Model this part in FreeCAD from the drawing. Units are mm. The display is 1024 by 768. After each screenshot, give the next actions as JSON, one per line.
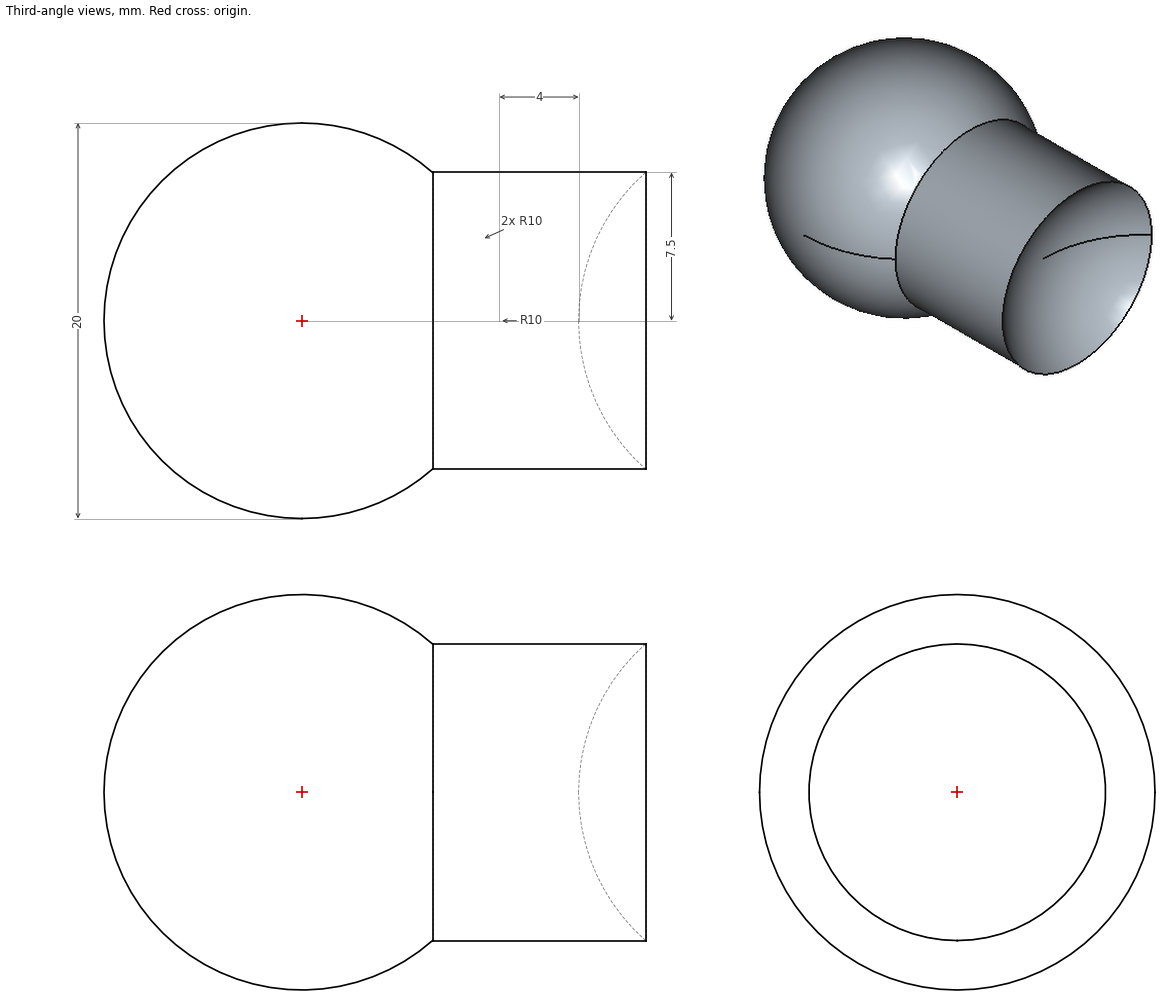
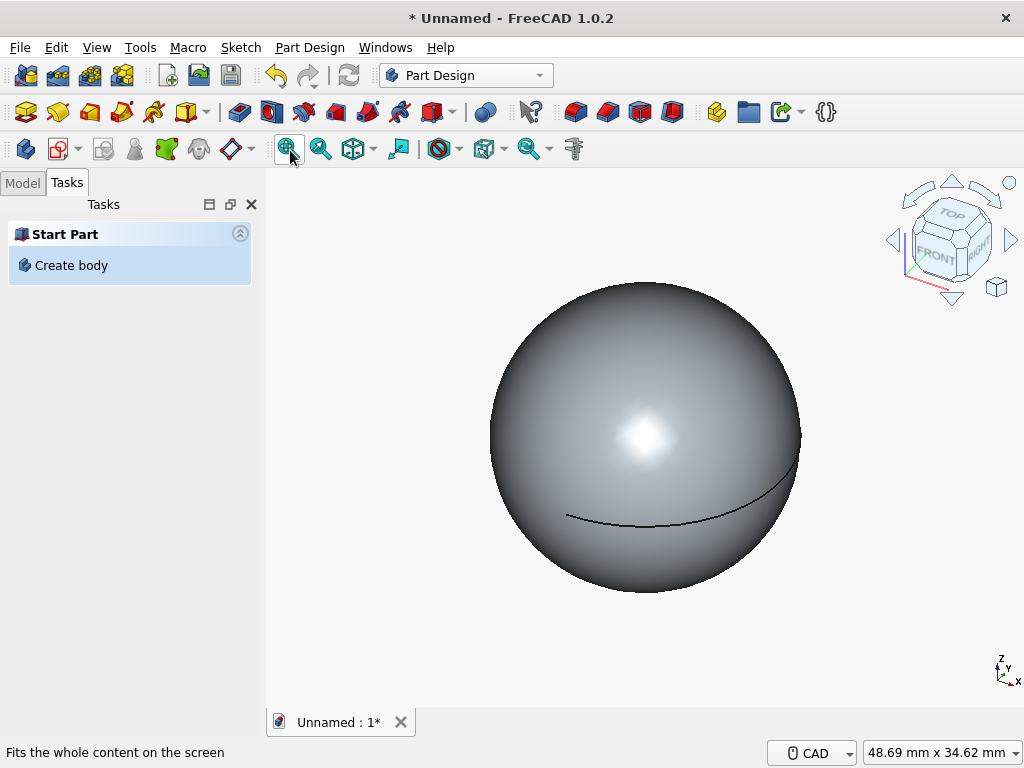
{"action": "left_click", "coordinate": [58, 150]}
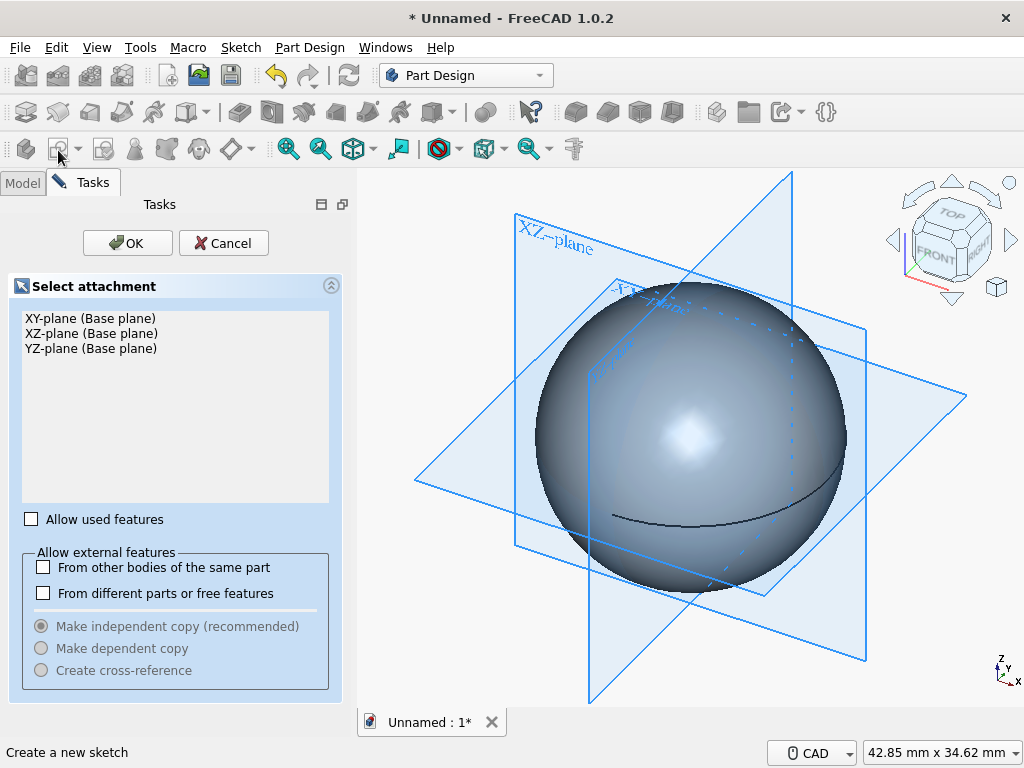
{"action": "left_click", "coordinate": [82, 318]}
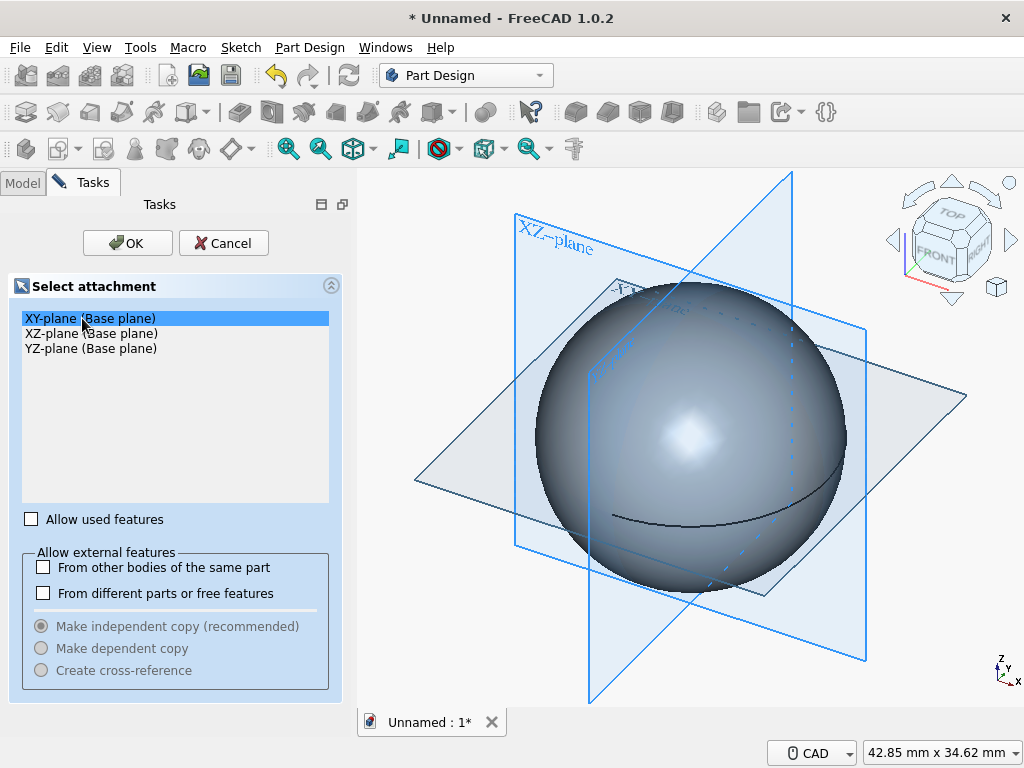
{"action": "left_click", "coordinate": [128, 243]}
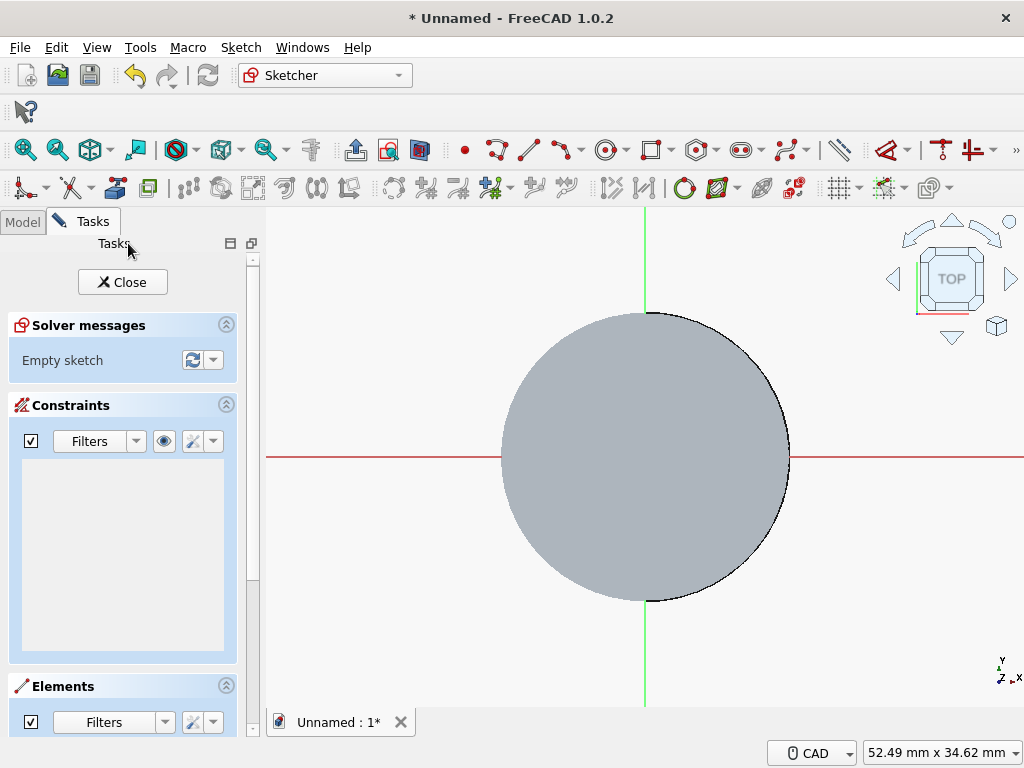
{"action": "key", "text": "q s"}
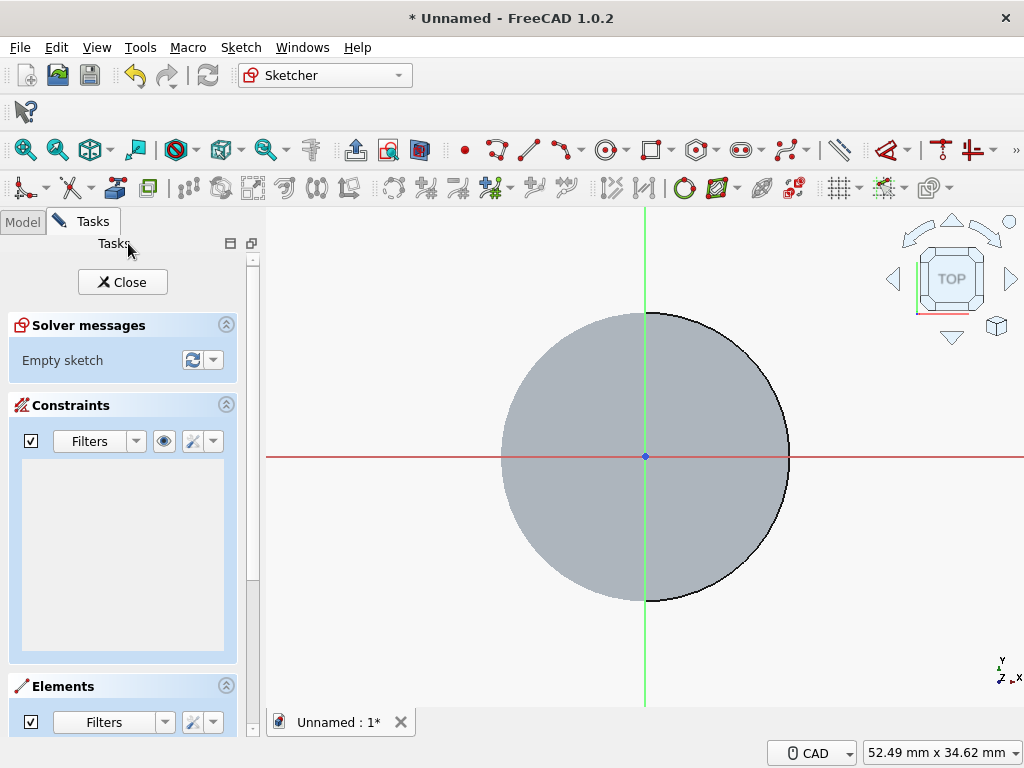
{"action": "scroll", "coordinate": [294, 679], "scroll_direction": "down", "scroll_amount": 1}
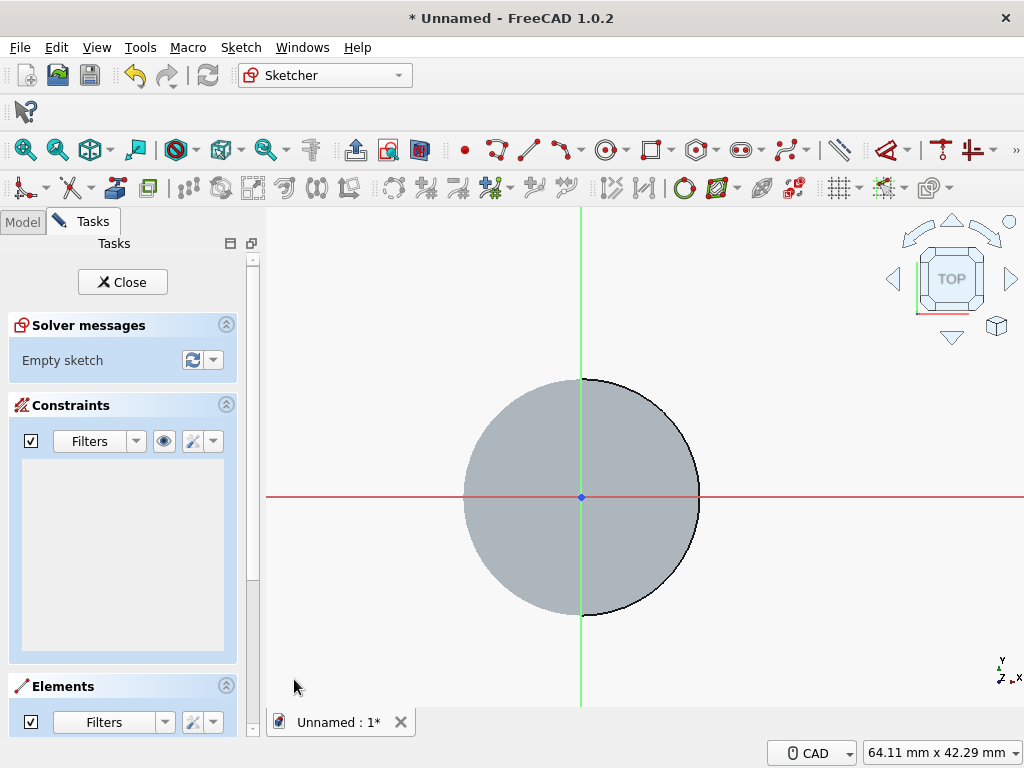
{"action": "scroll", "coordinate": [815, 448], "scroll_direction": "up", "scroll_amount": 3}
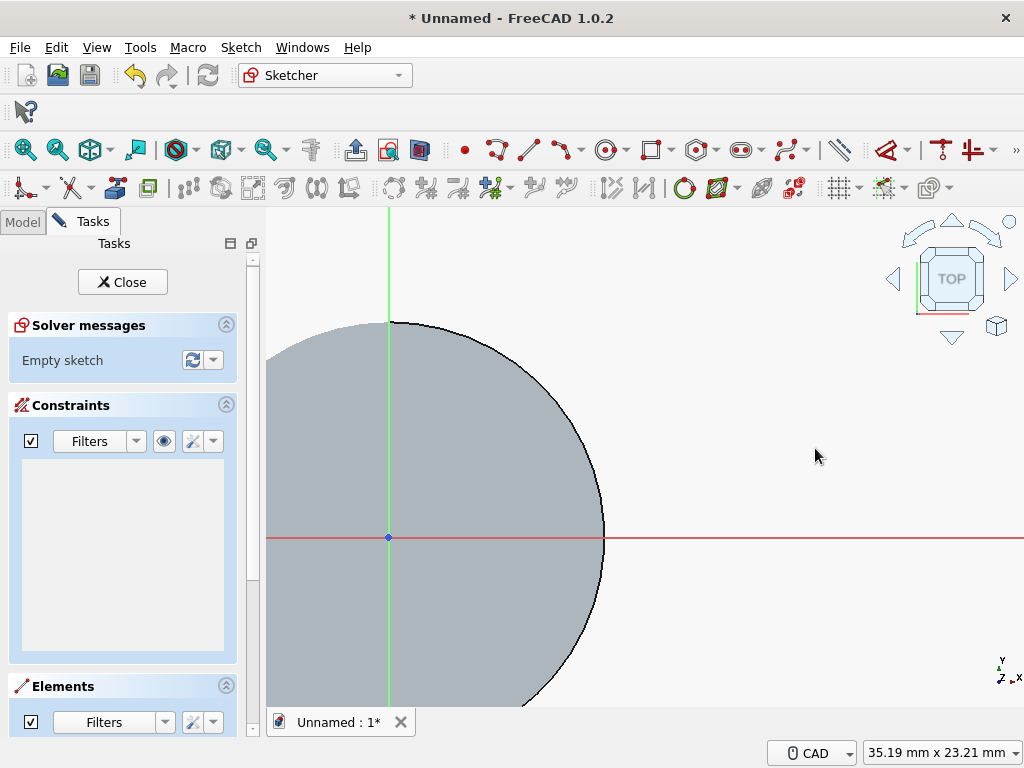
{"action": "key", "text": "g l"}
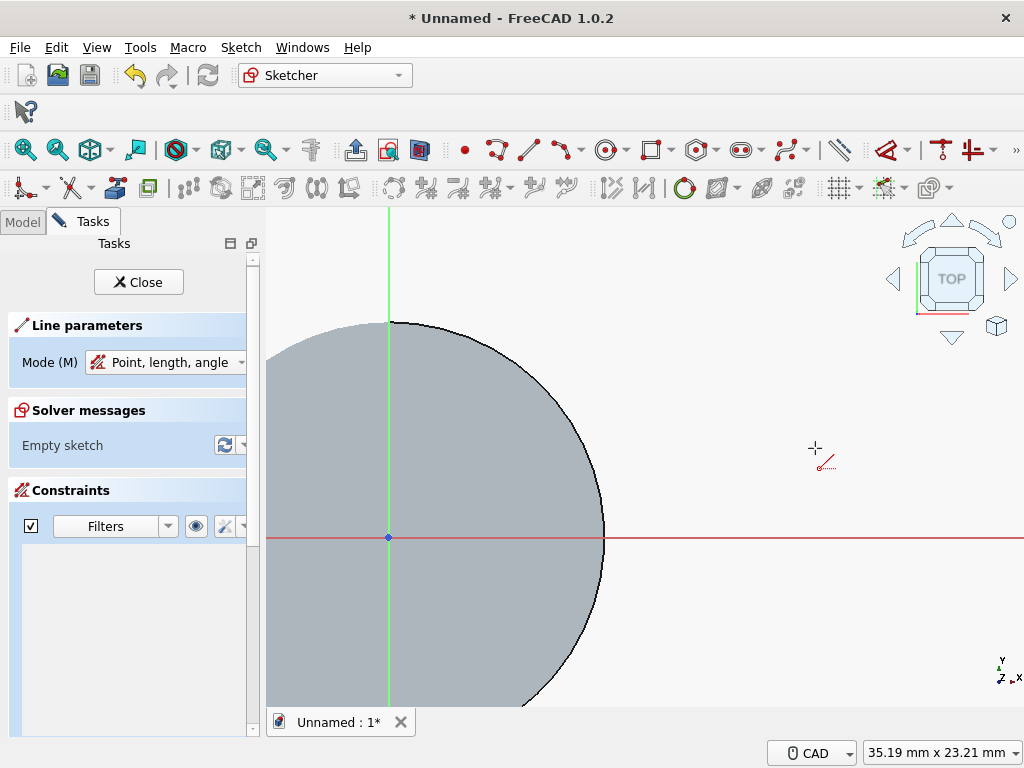
{"action": "left_click", "coordinate": [763, 376]}
{"action": "left_click", "coordinate": [531, 376]}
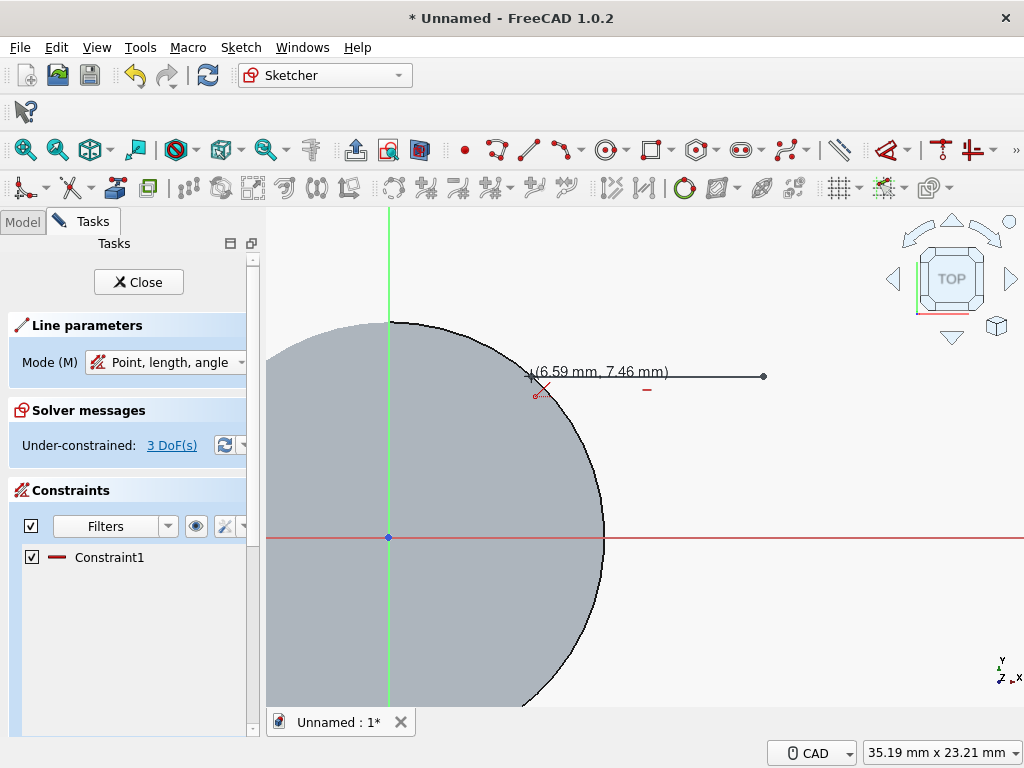
{"action": "left_click", "coordinate": [604, 538]}
{"action": "left_click", "coordinate": [691, 529]}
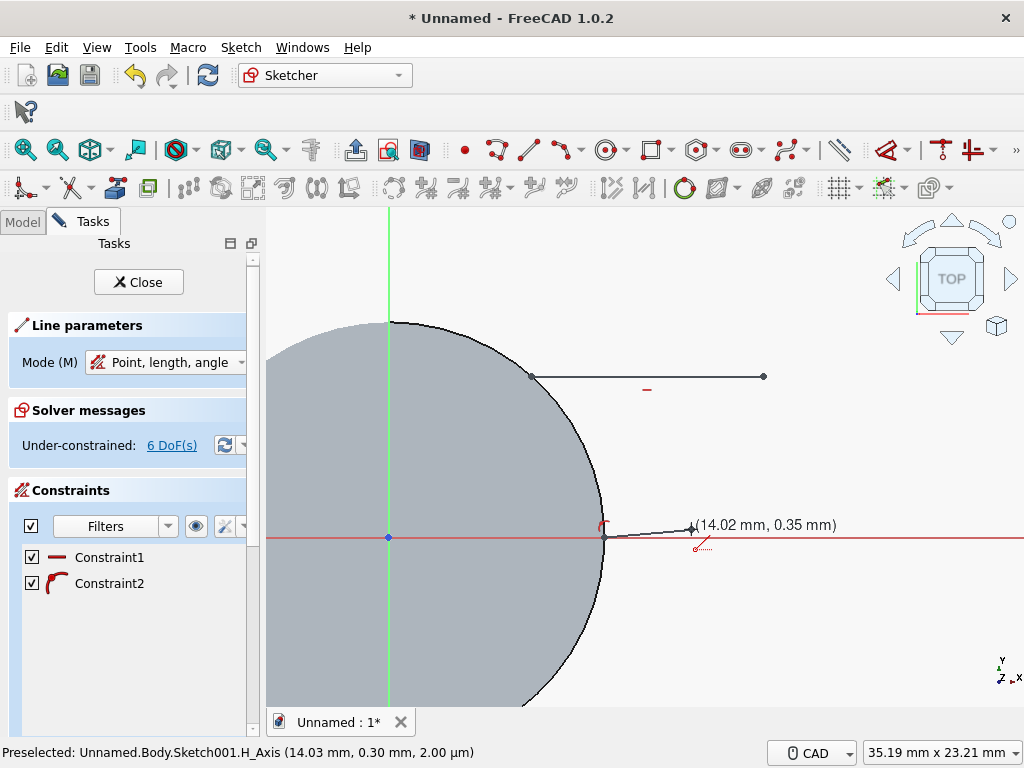
{"action": "left_click", "coordinate": [562, 150]}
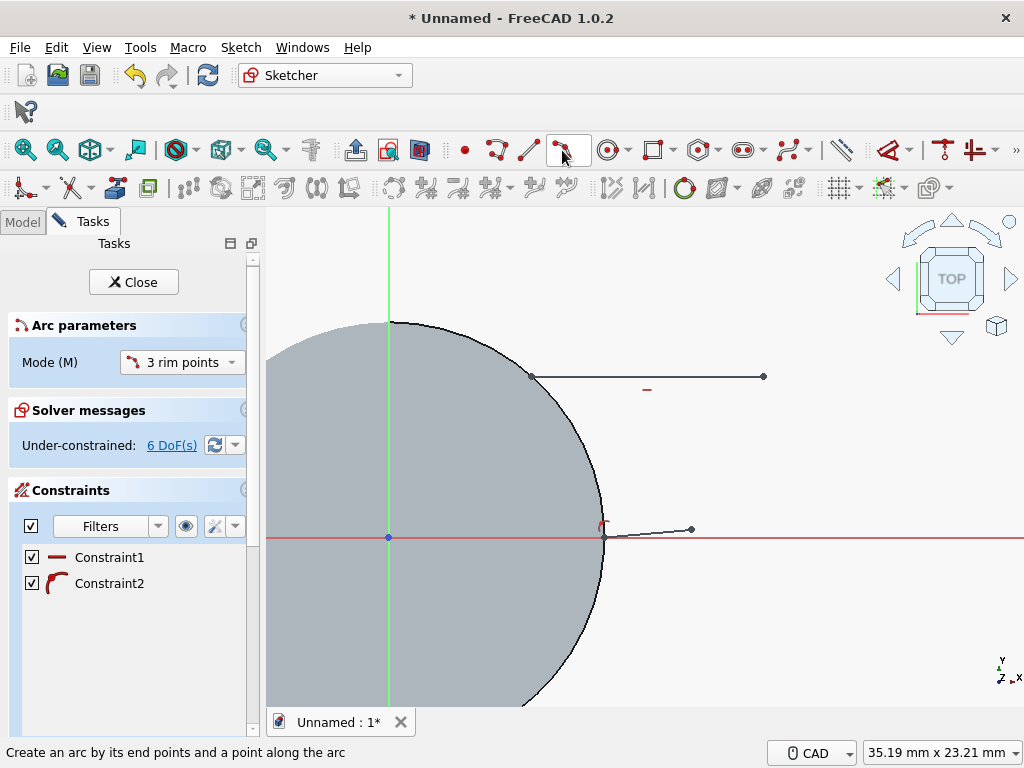
{"action": "left_click", "coordinate": [531, 377]}
{"action": "left_click", "coordinate": [604, 538]}
{"action": "left_click", "coordinate": [585, 449]}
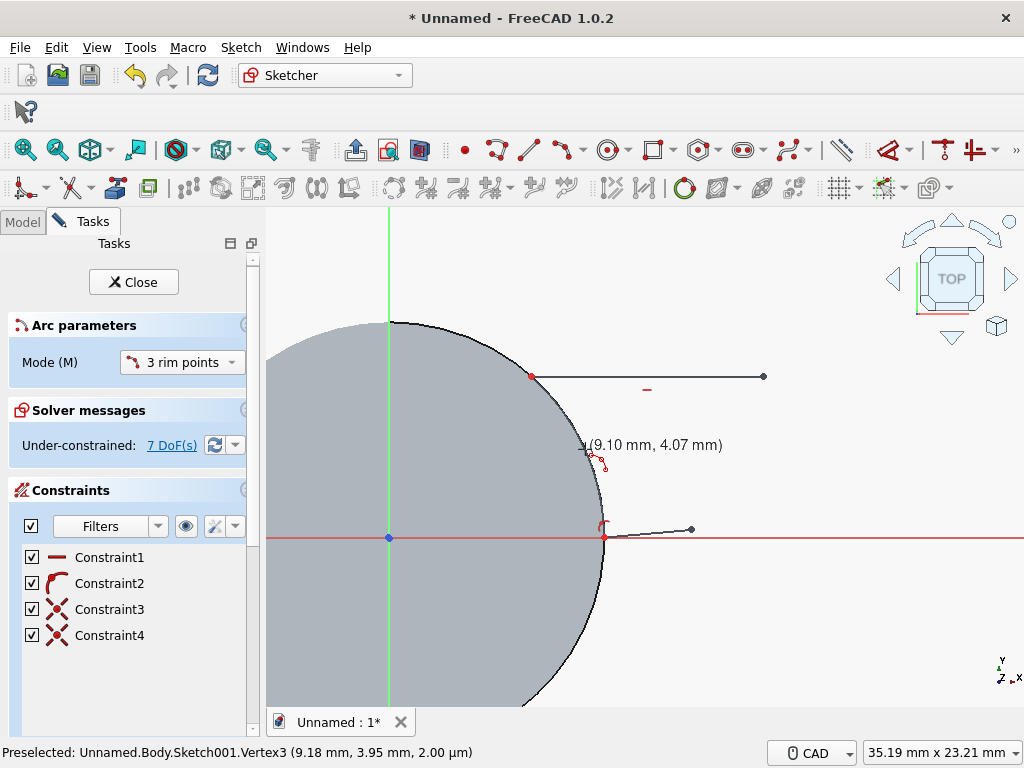
{"action": "left_click", "coordinate": [691, 530]}
{"action": "left_click", "coordinate": [763, 377]}
{"action": "left_click", "coordinate": [710, 449]}
{"action": "key", "text": "Escape"}